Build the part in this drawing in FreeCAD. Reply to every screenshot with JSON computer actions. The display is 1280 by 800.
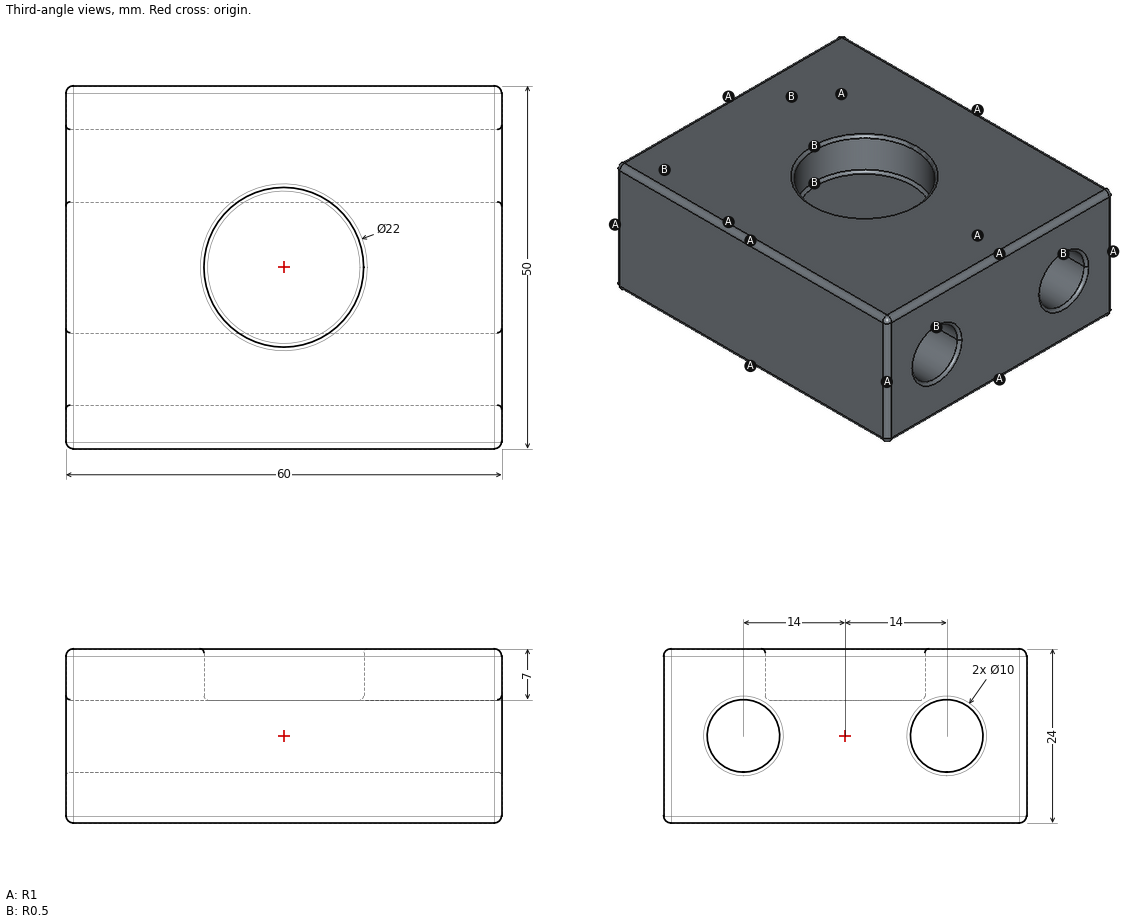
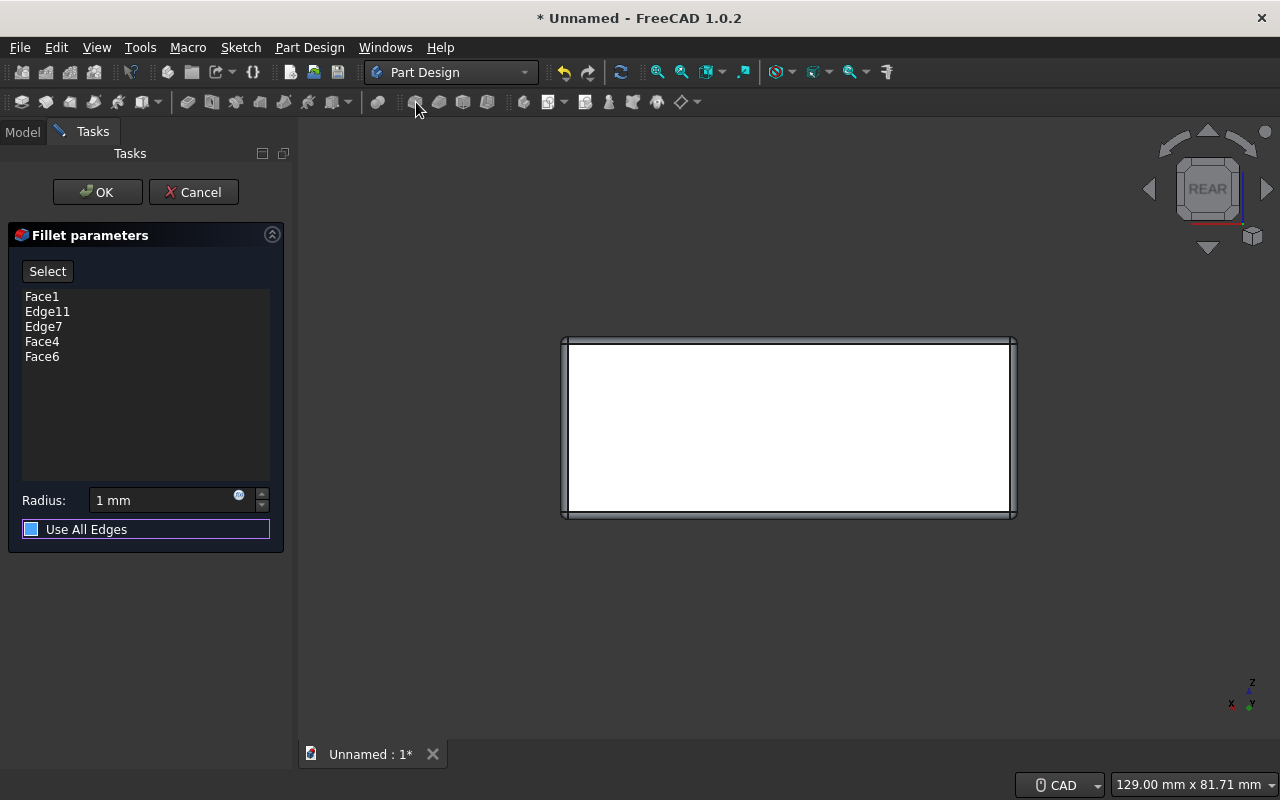
{"action": "left_click", "coordinate": [98, 192]}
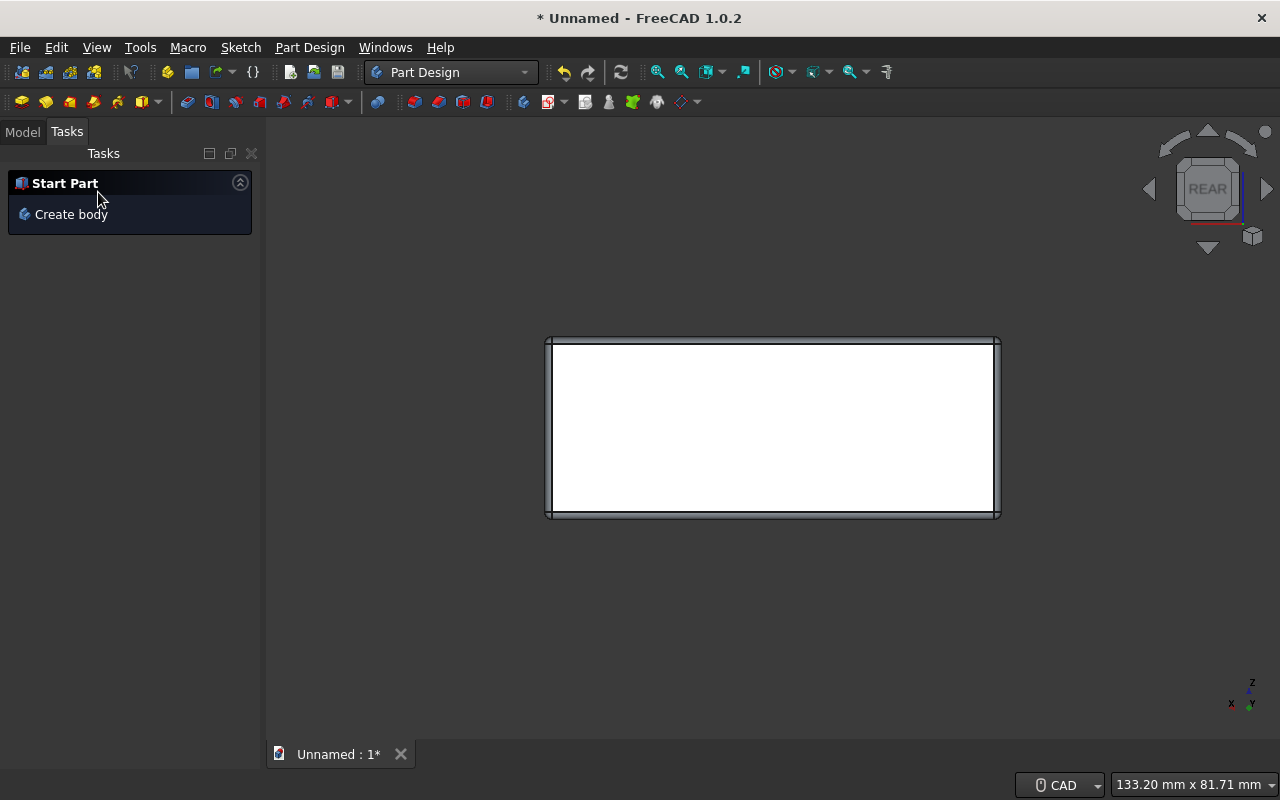
{"action": "left_click", "coordinate": [658, 72]}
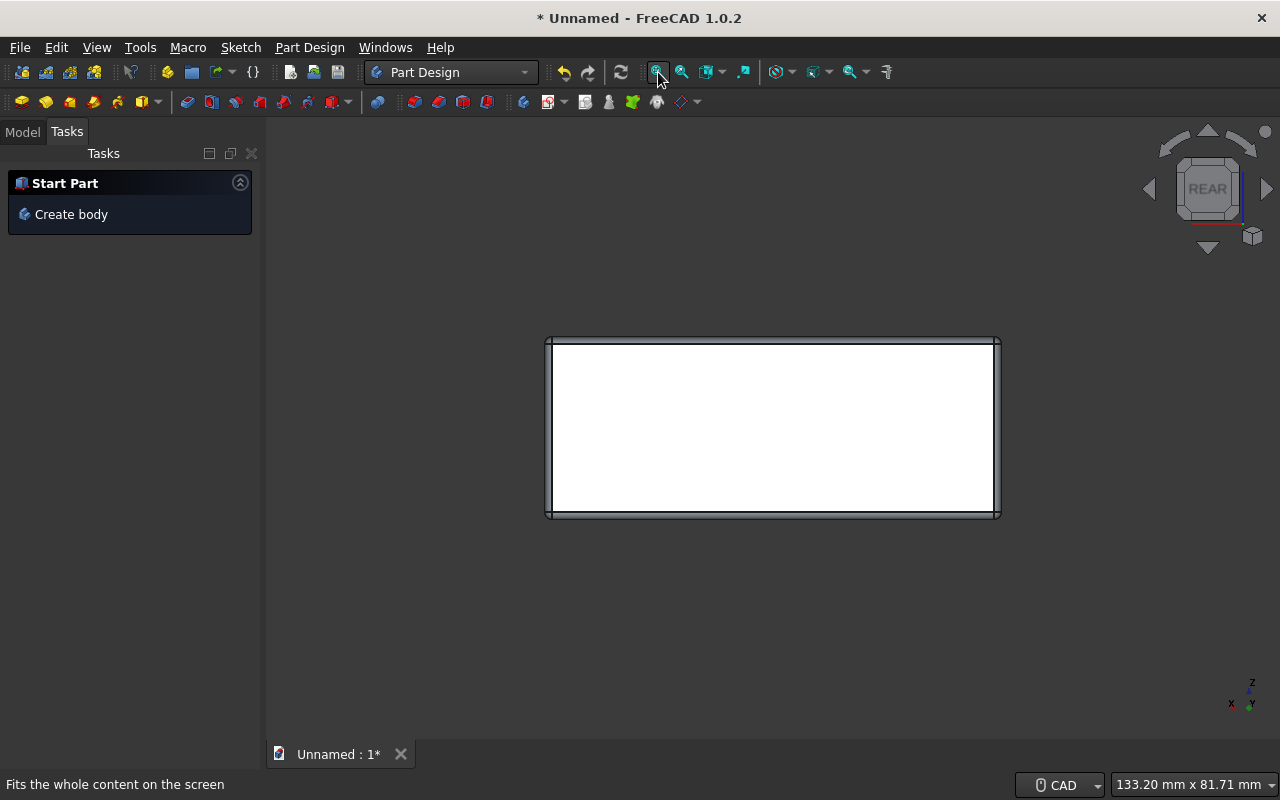
{"action": "key", "text": "0"}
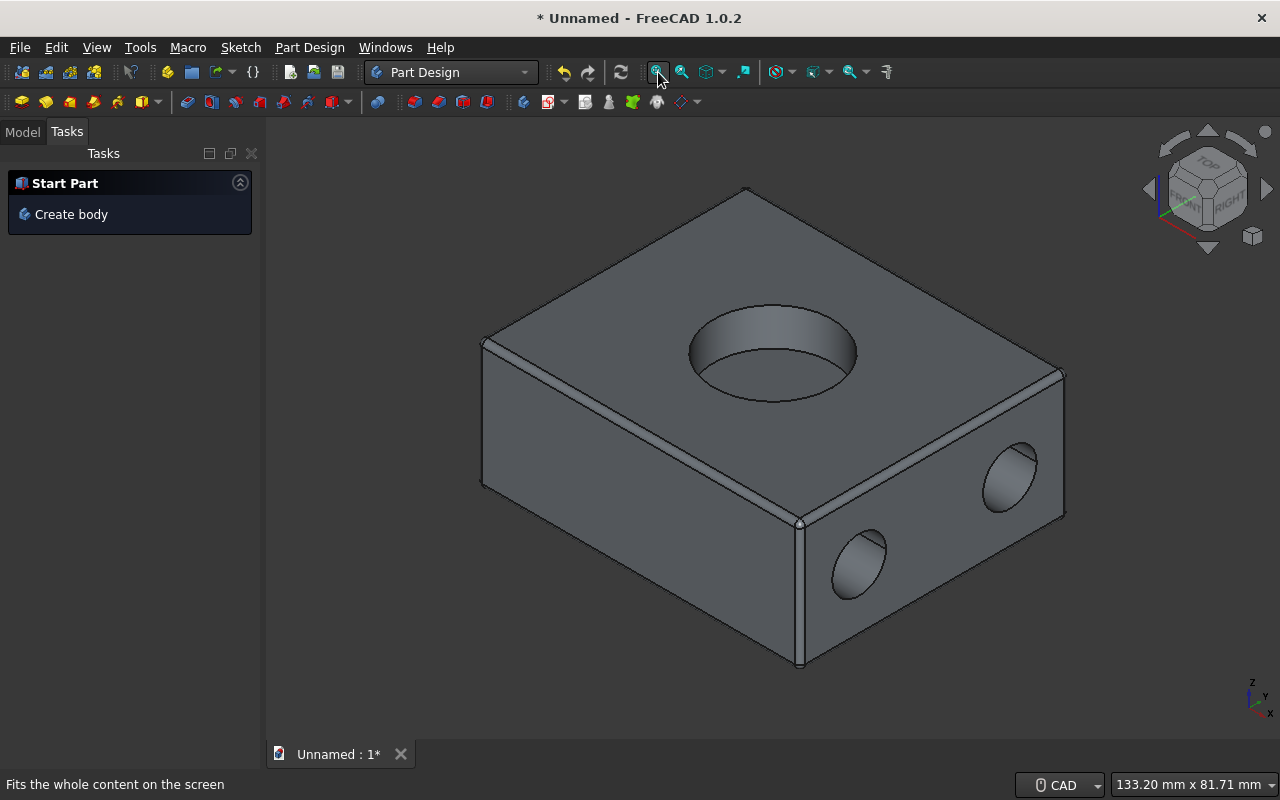
{"action": "left_click", "coordinate": [714, 318]}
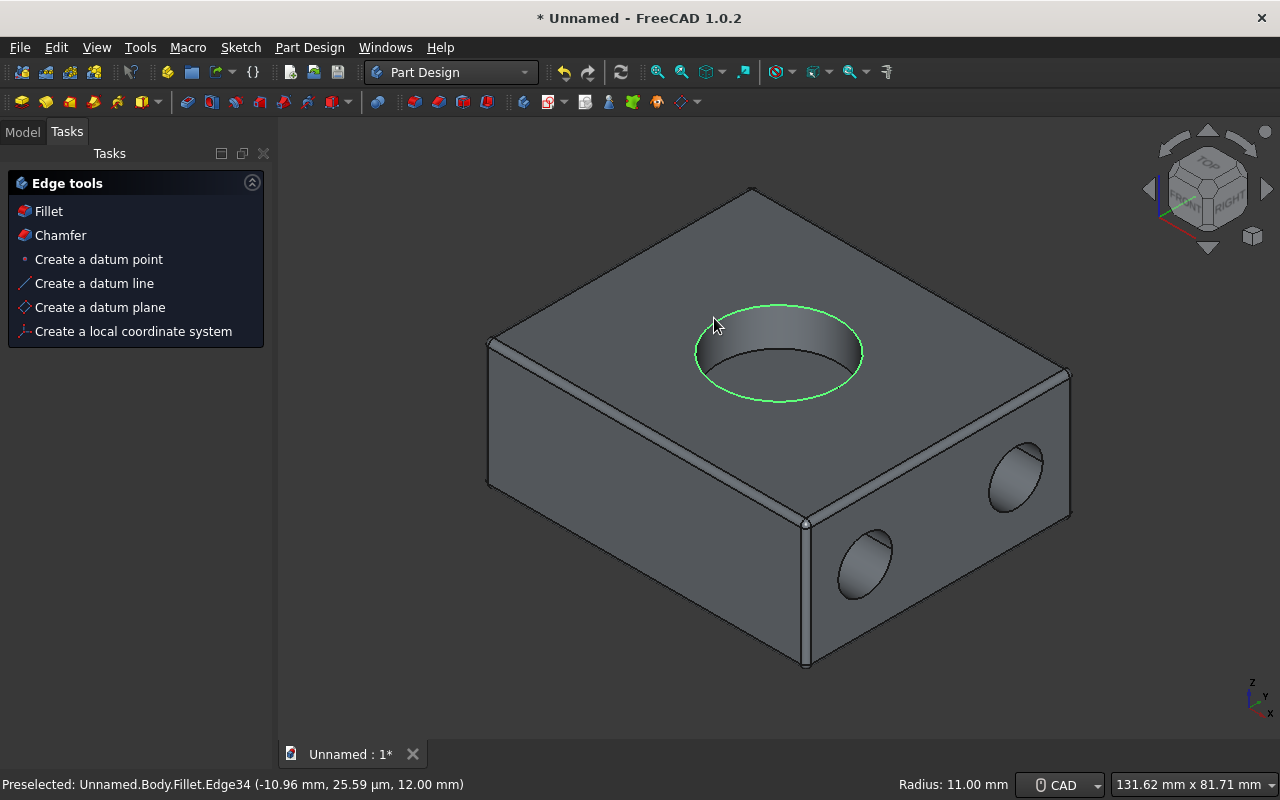
{"action": "left_click", "coordinate": [1008, 511], "text": "ctrl"}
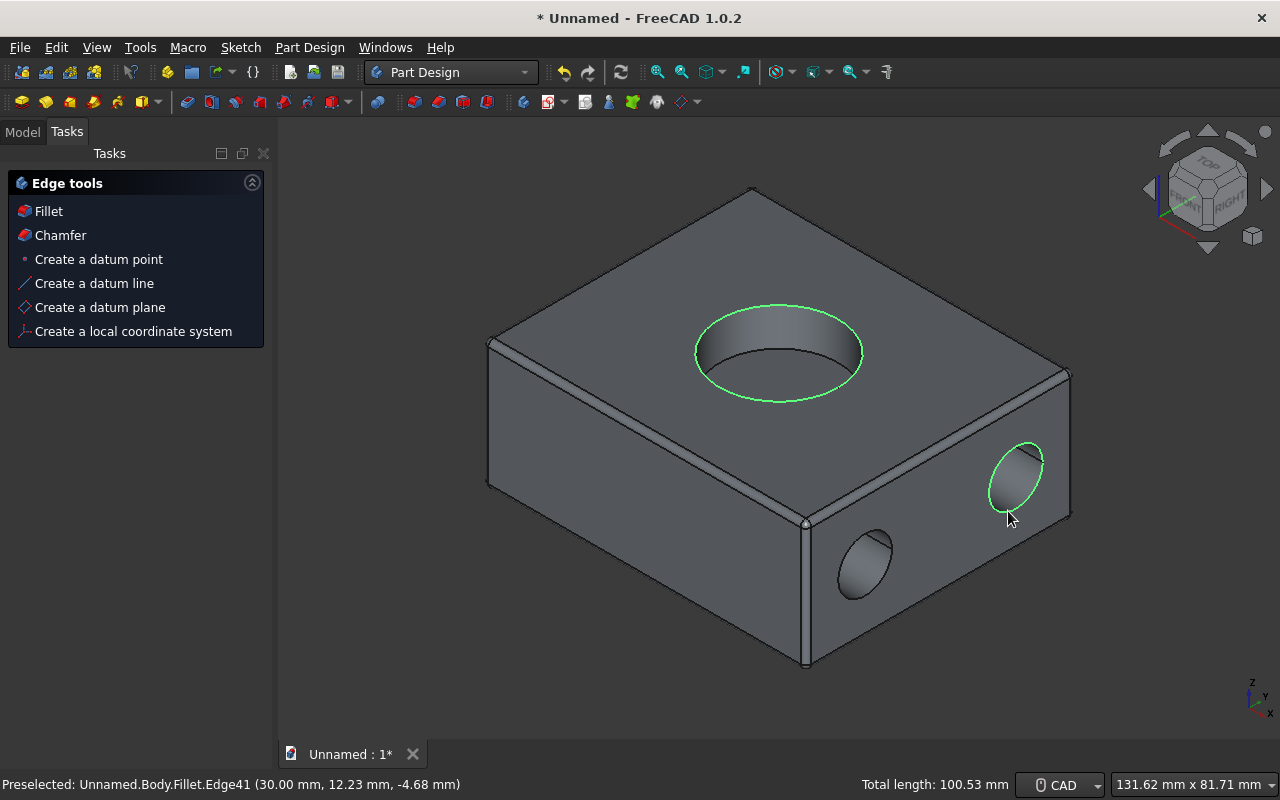
{"action": "left_click", "coordinate": [857, 598], "text": "ctrl"}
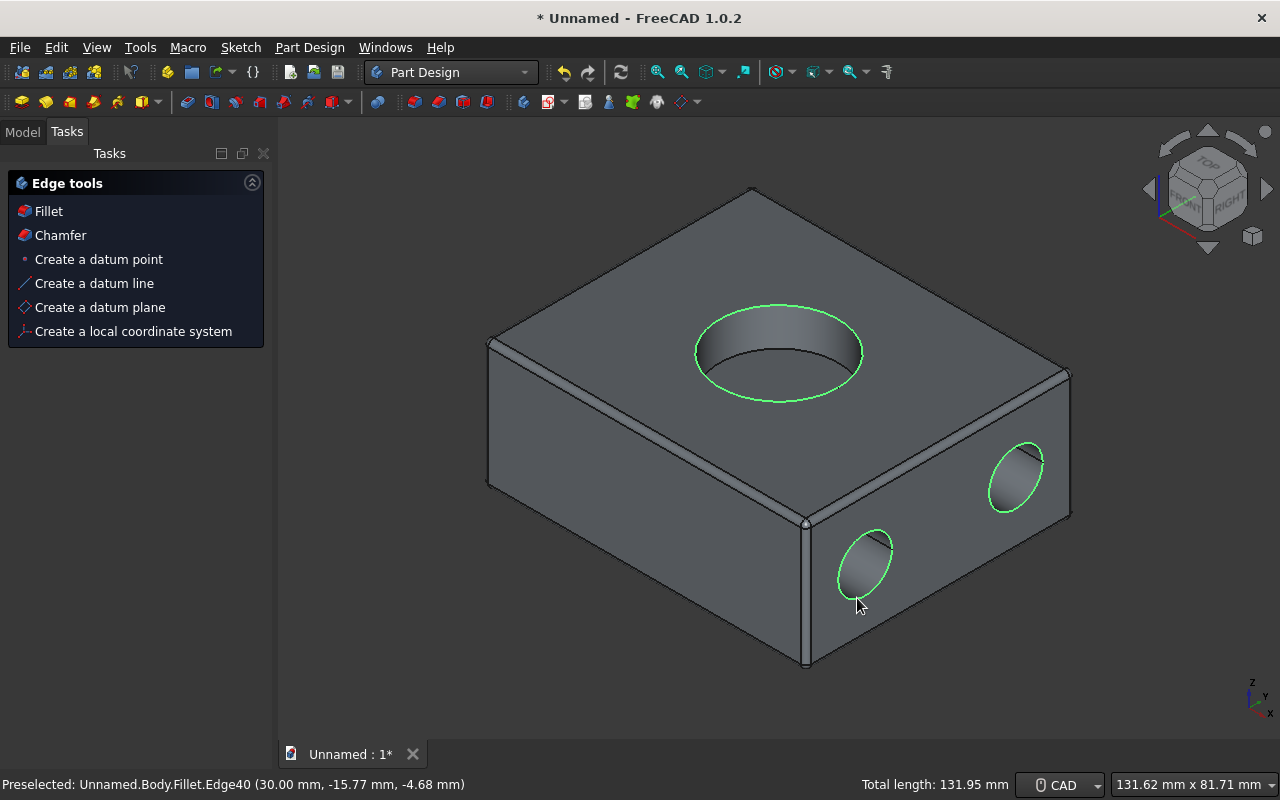
{"action": "key", "text": "2"}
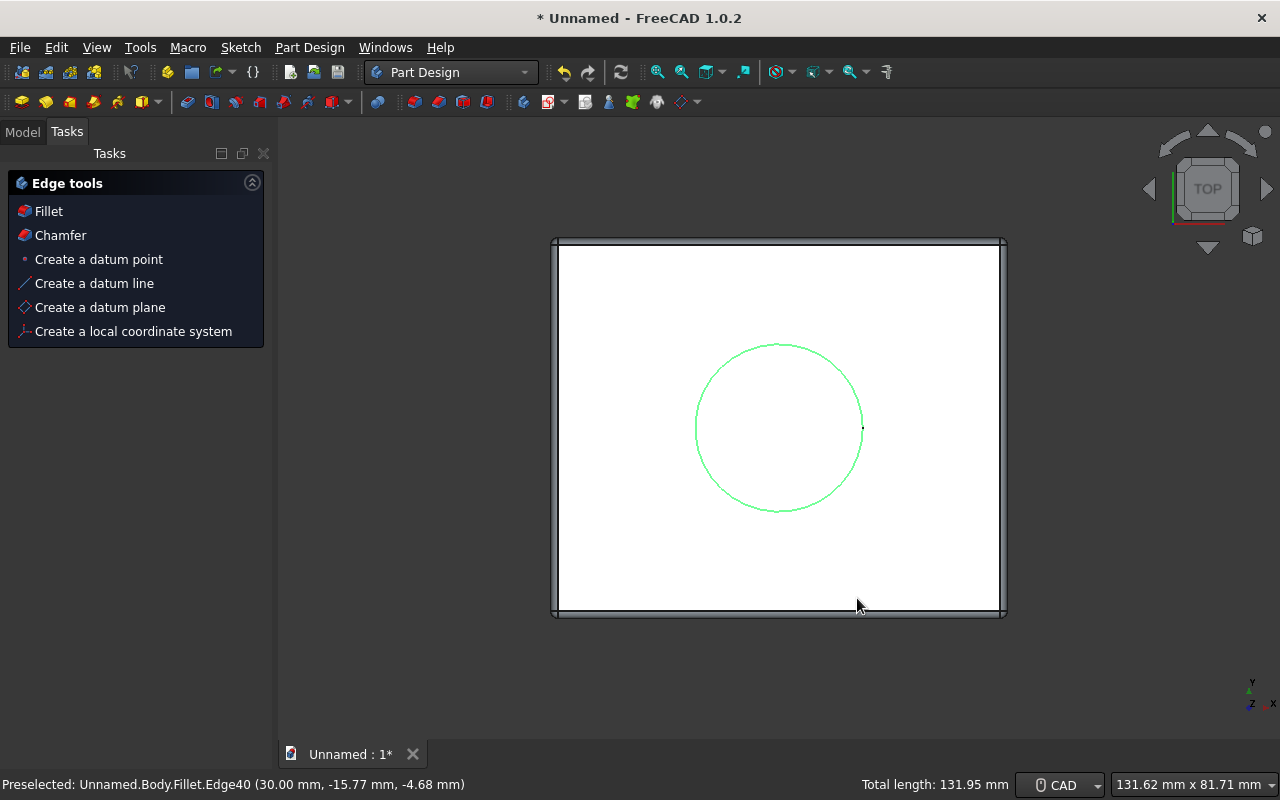
{"action": "key", "text": "1"}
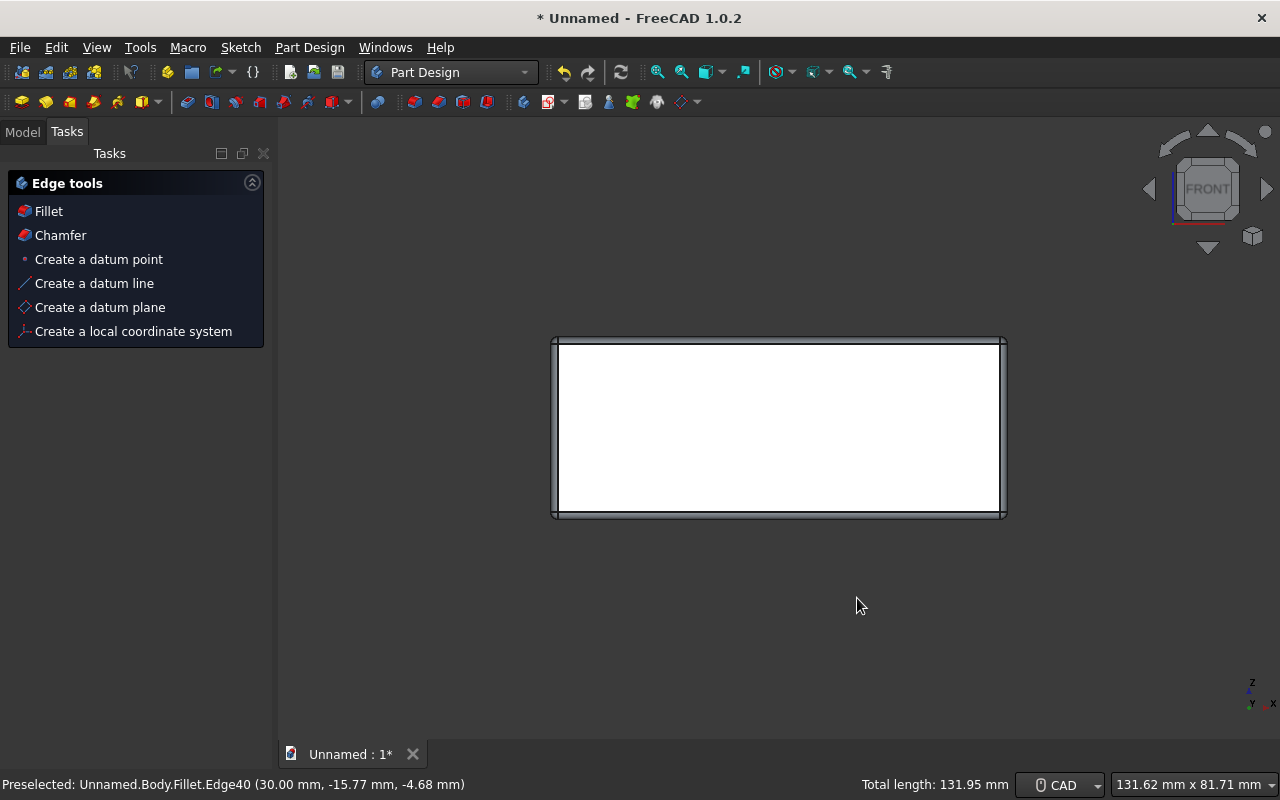
{"action": "key", "text": "3"}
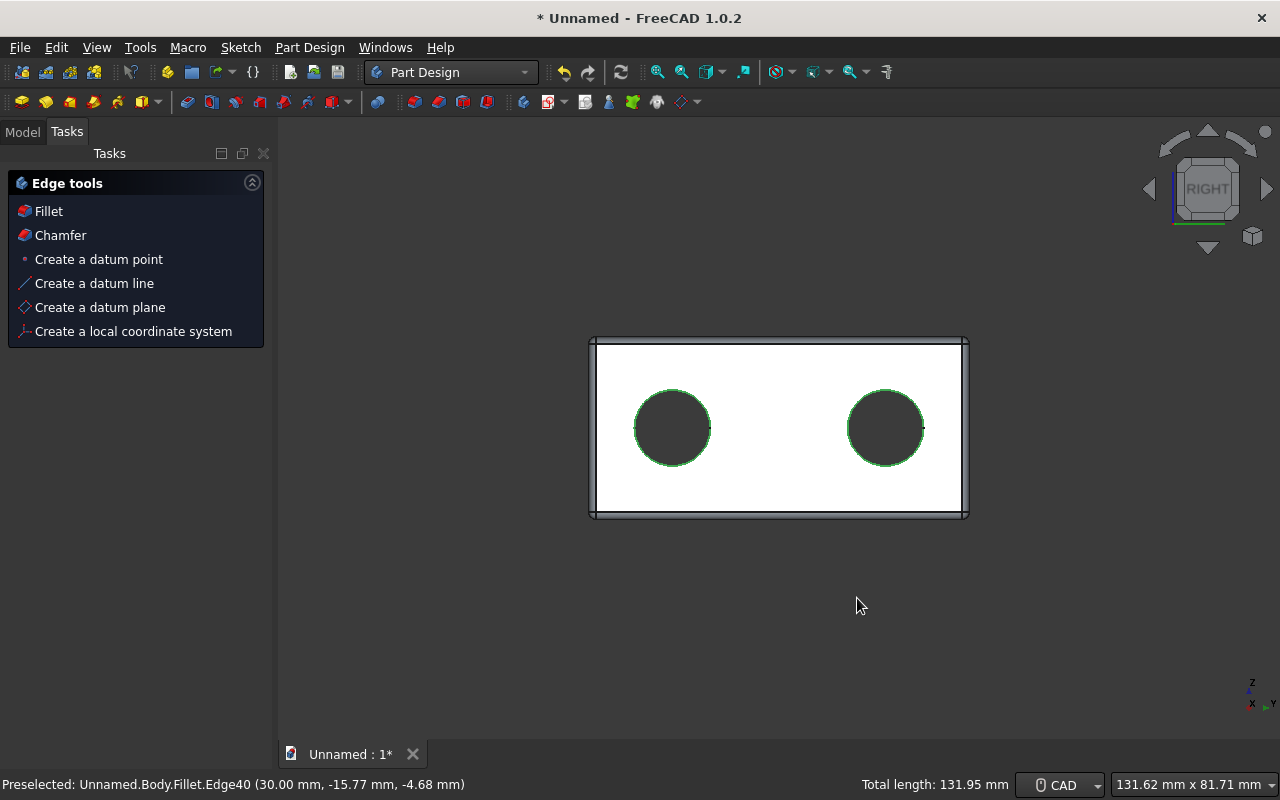
{"action": "left_click", "coordinate": [658, 72]}